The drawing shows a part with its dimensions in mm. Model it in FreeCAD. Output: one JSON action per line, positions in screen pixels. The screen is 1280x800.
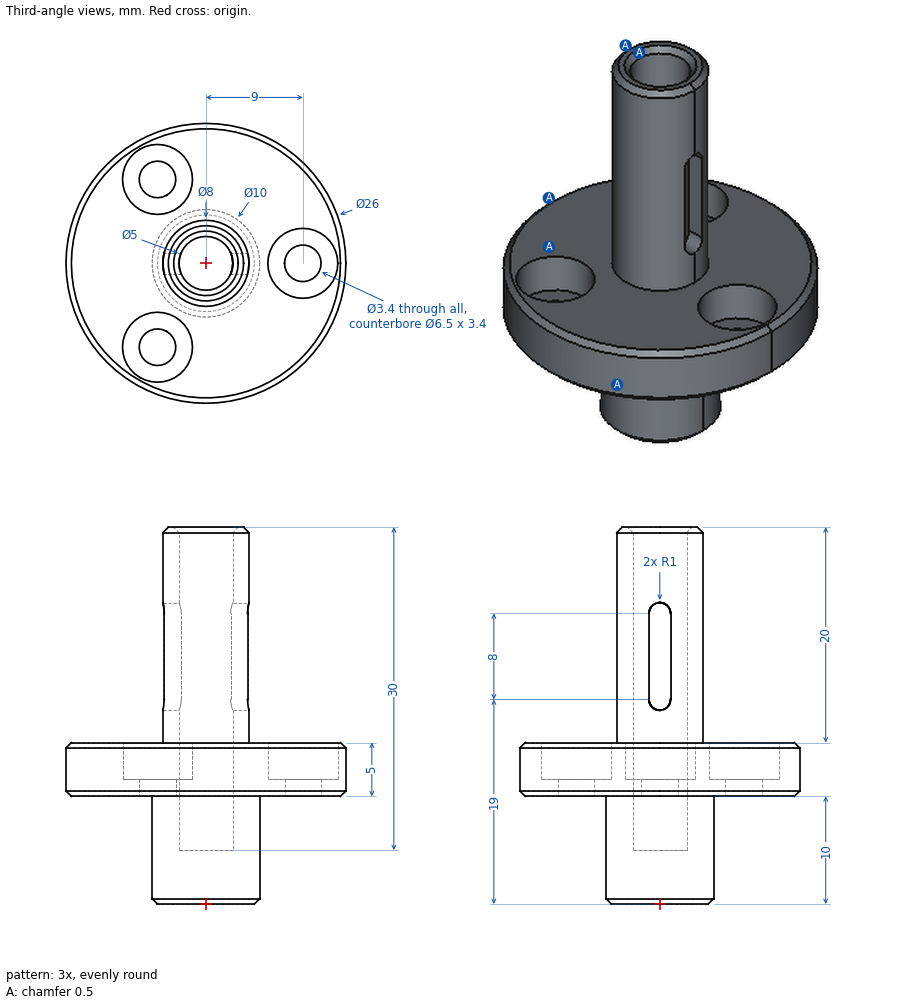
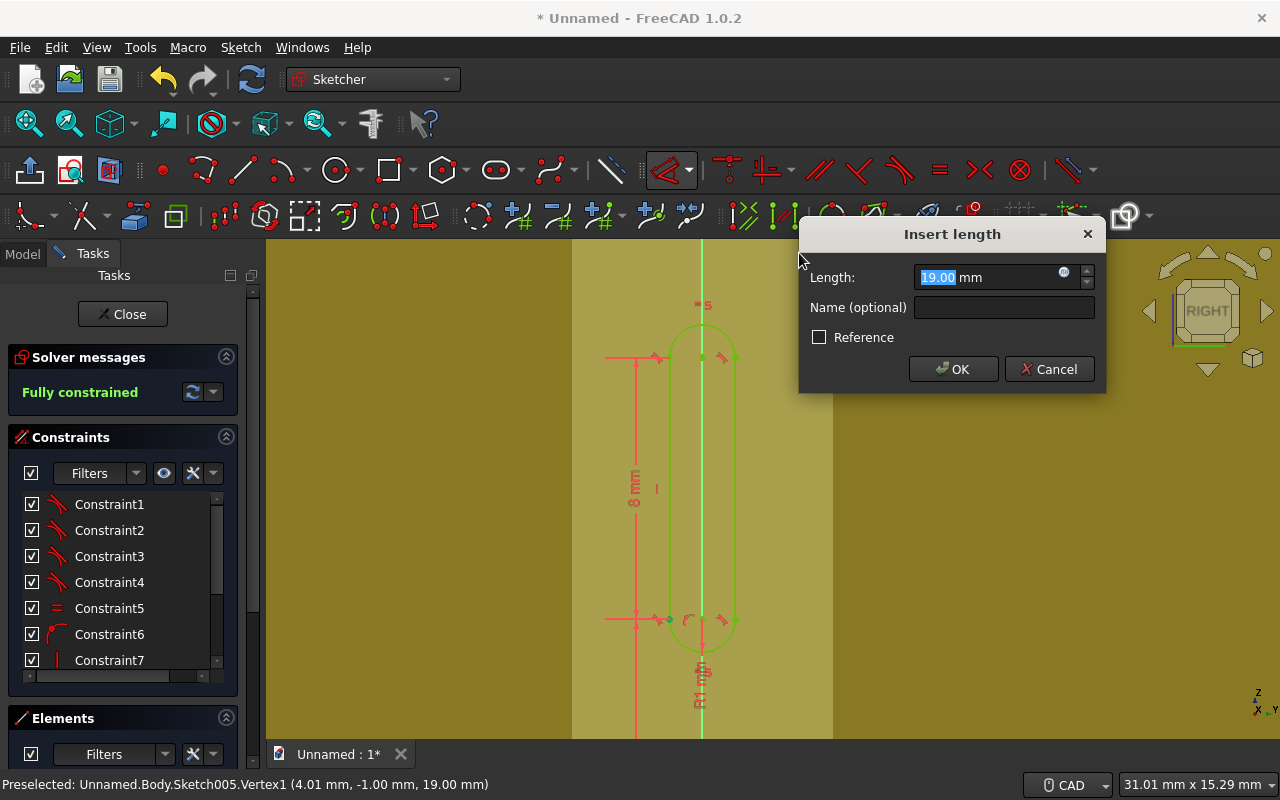
{"action": "type", "text": "19"}
{"action": "key", "text": "Return"}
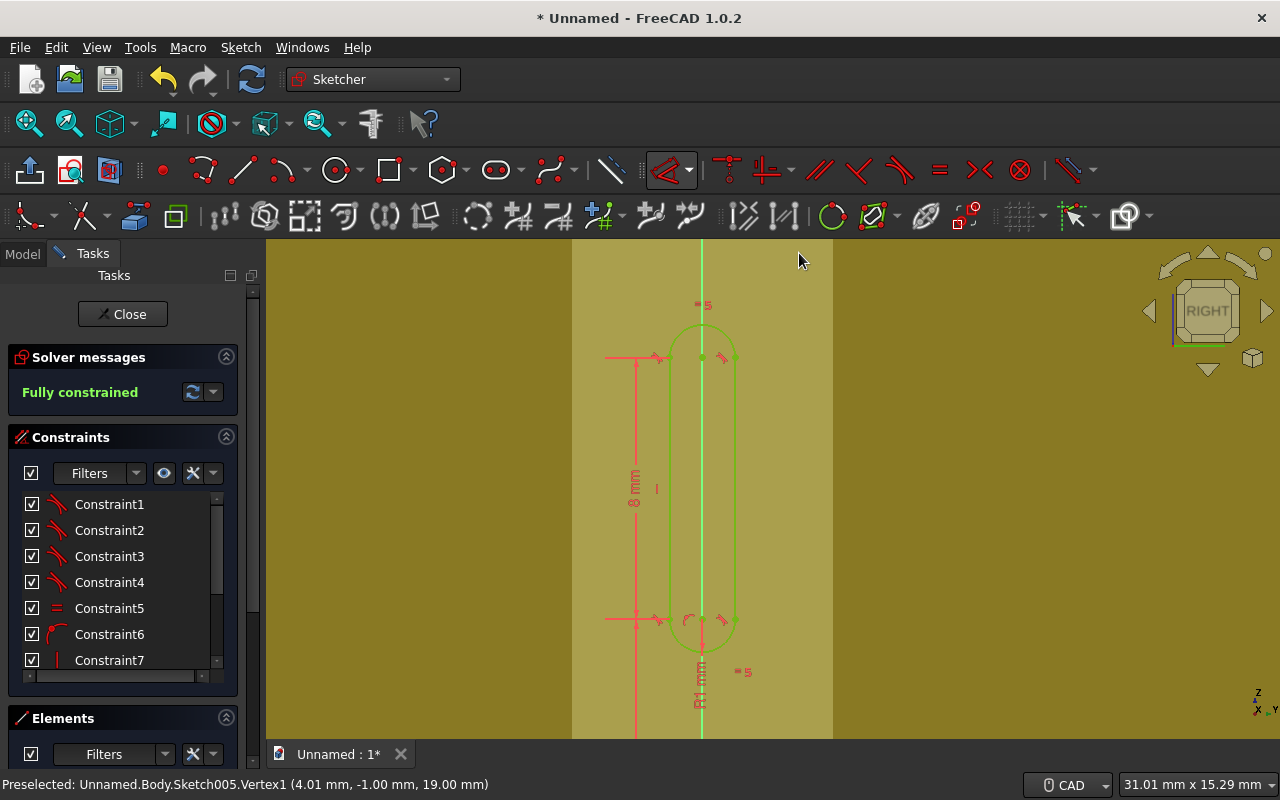
{"action": "left_click", "coordinate": [123, 314]}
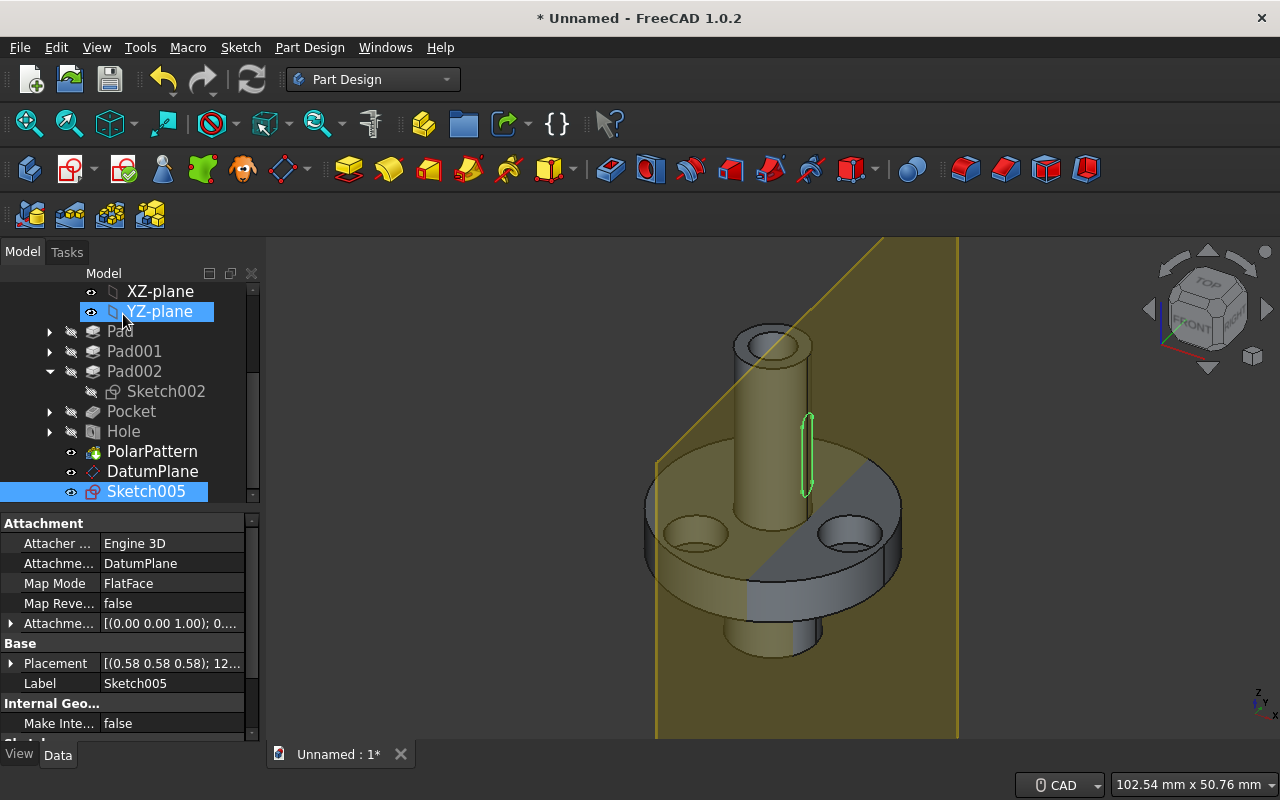
{"action": "left_click", "coordinate": [612, 170]}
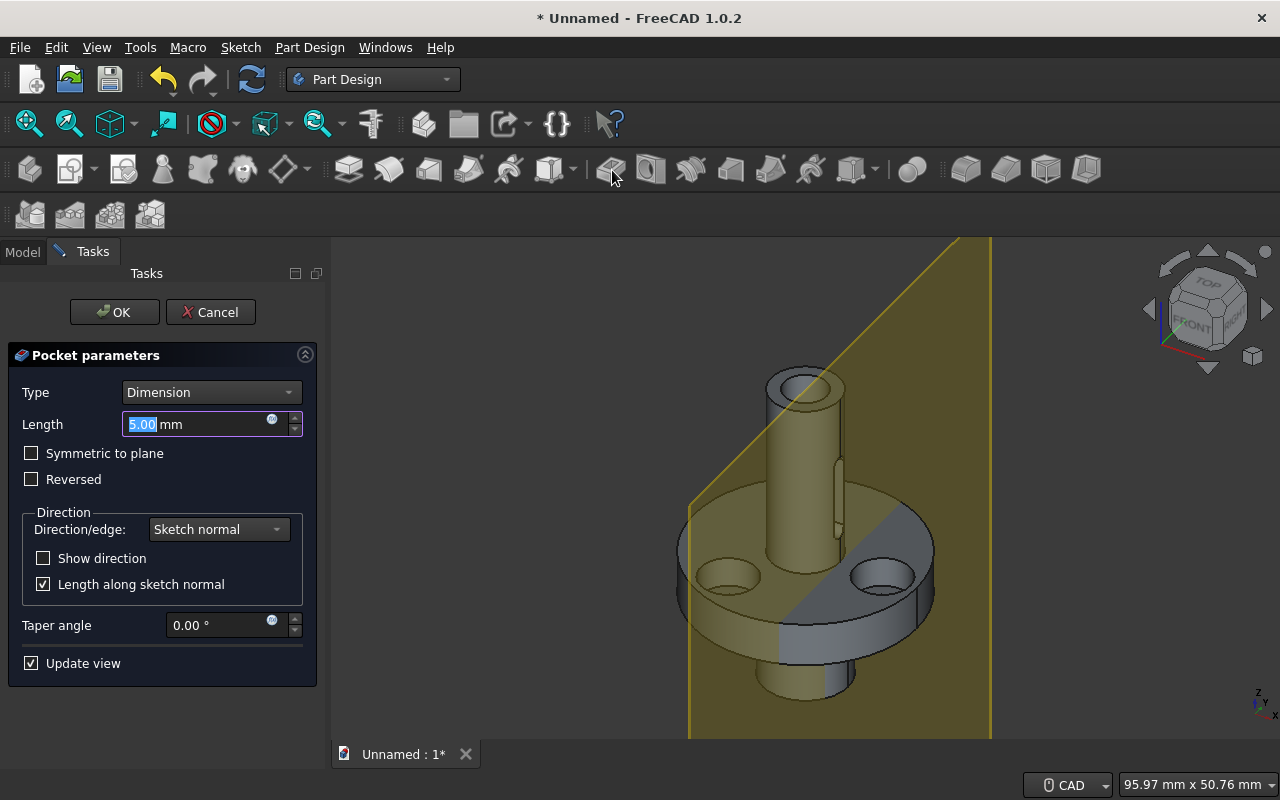
{"action": "left_click", "coordinate": [212, 392]}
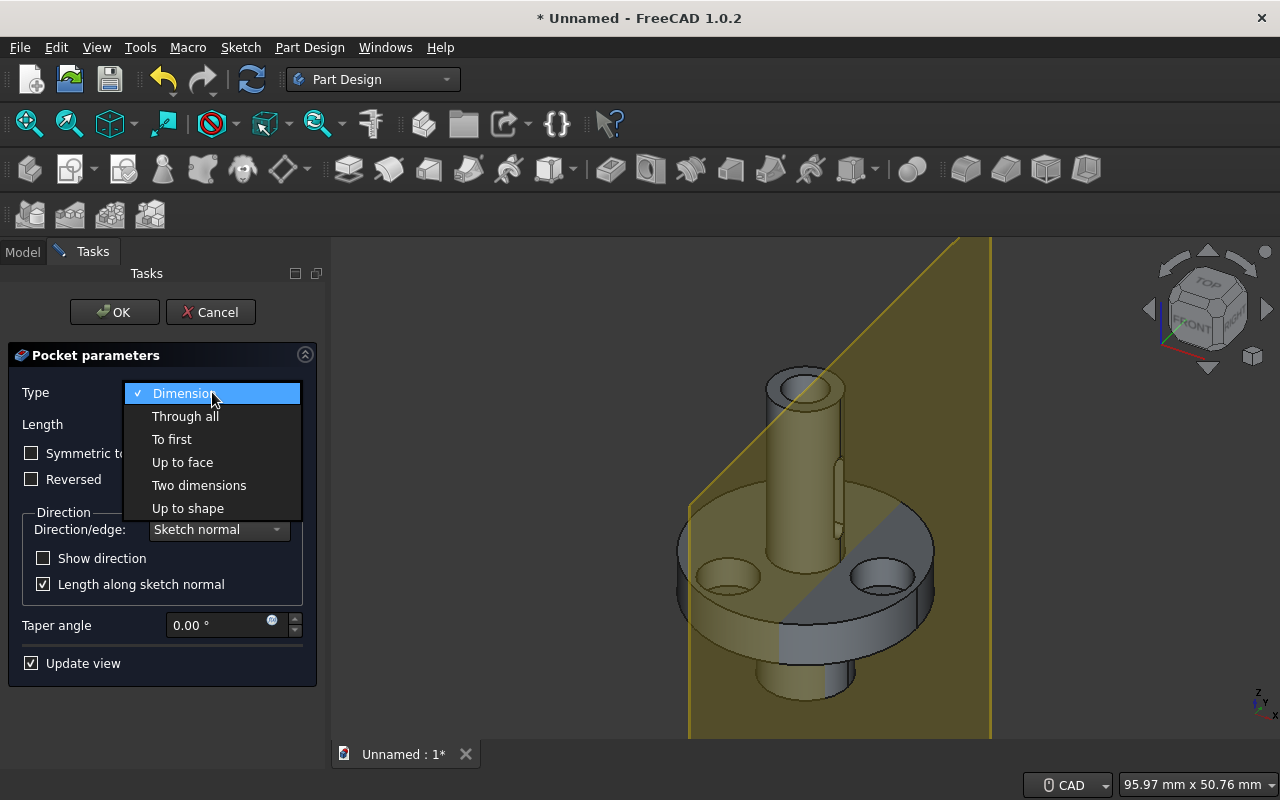
{"action": "left_click", "coordinate": [212, 416]}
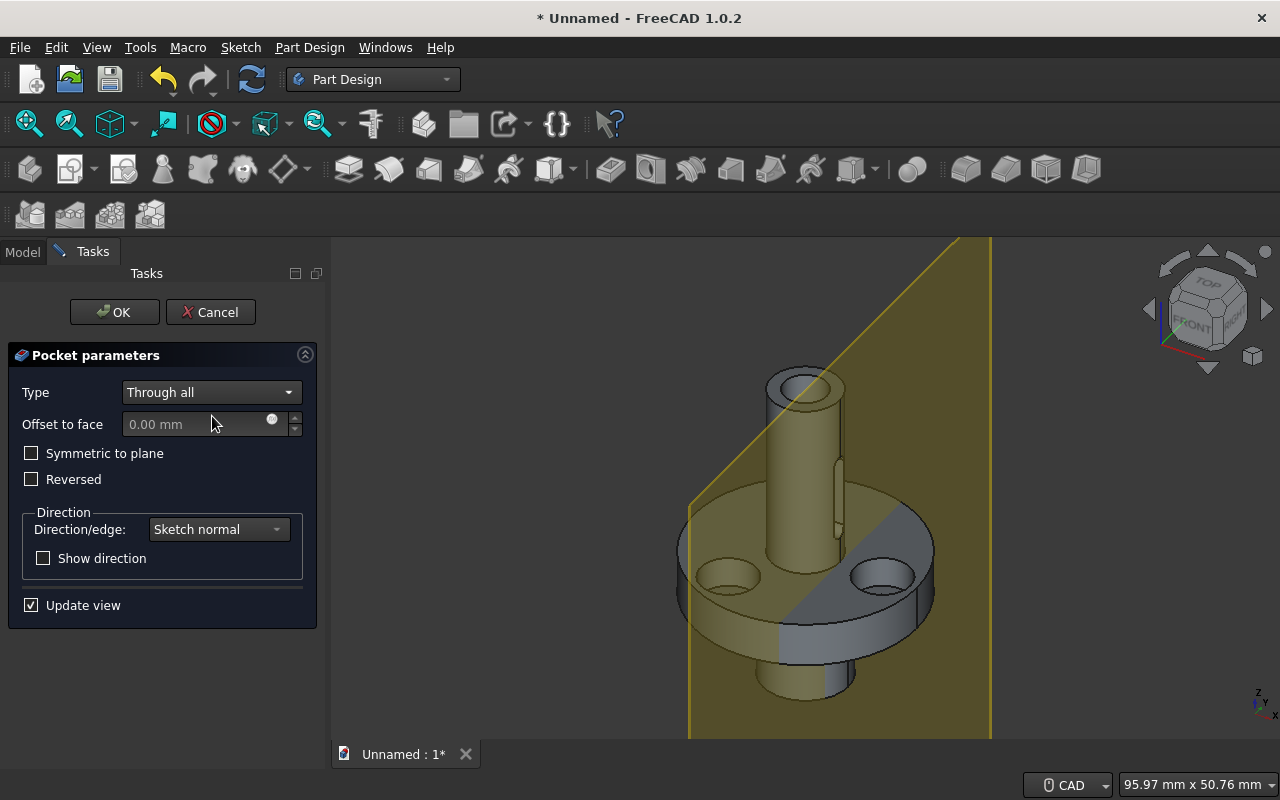
{"action": "left_click", "coordinate": [115, 312]}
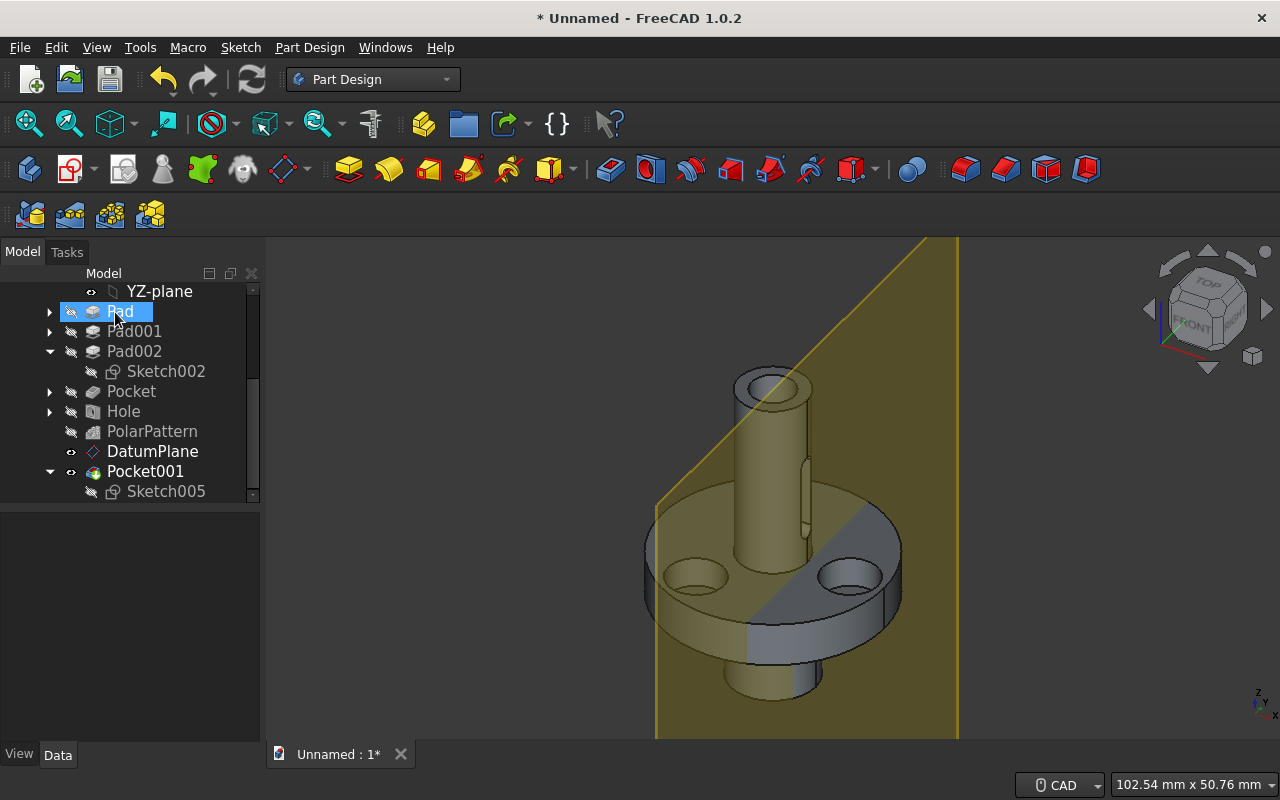
{"action": "left_click", "coordinate": [116, 452]}
{"action": "key", "text": "space"}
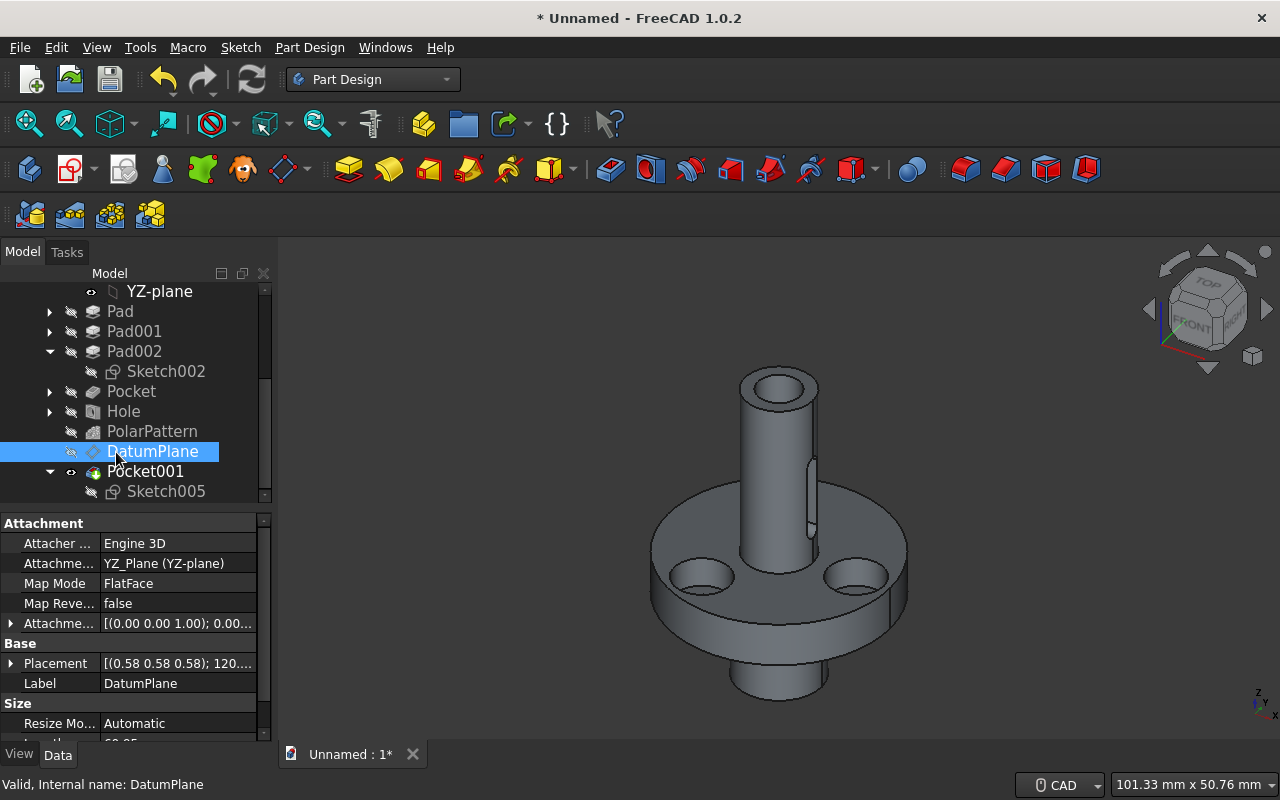
{"action": "left_click", "coordinate": [30, 124]}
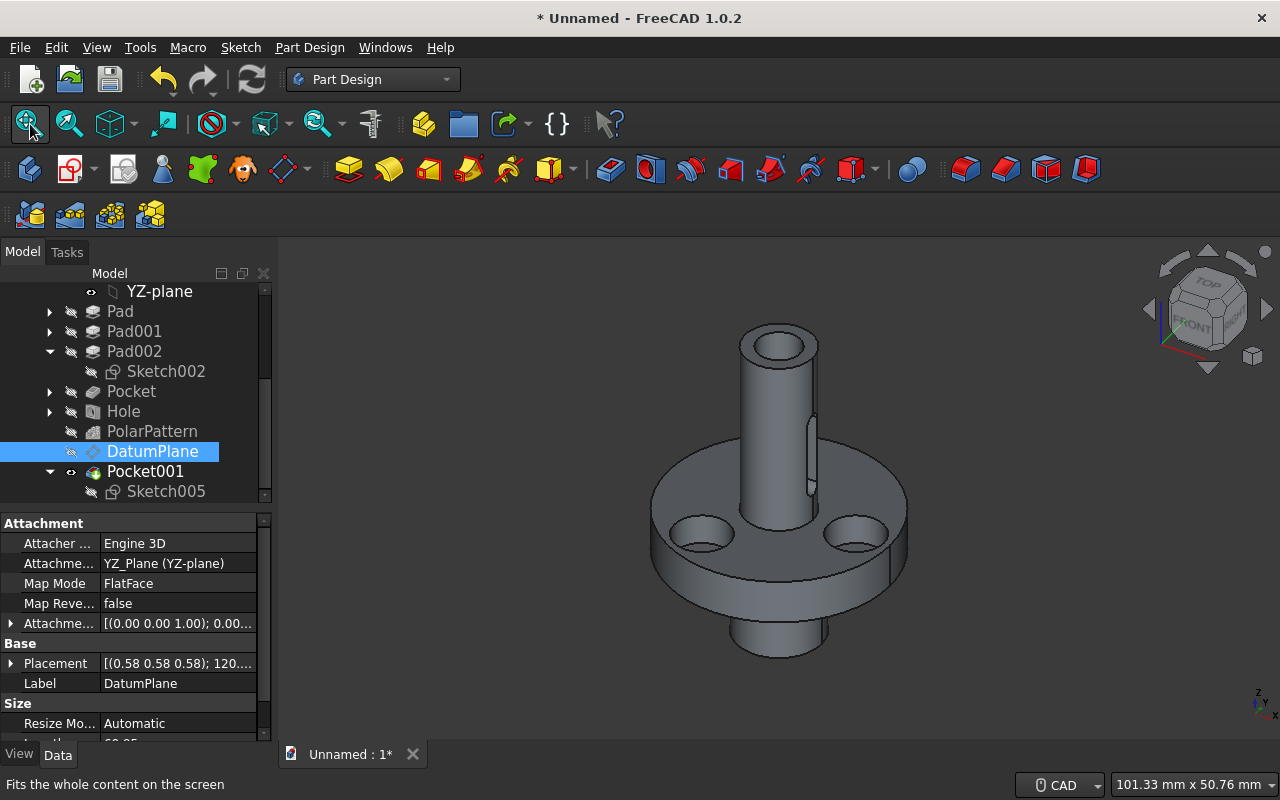
{"action": "left_click", "coordinate": [740, 348]}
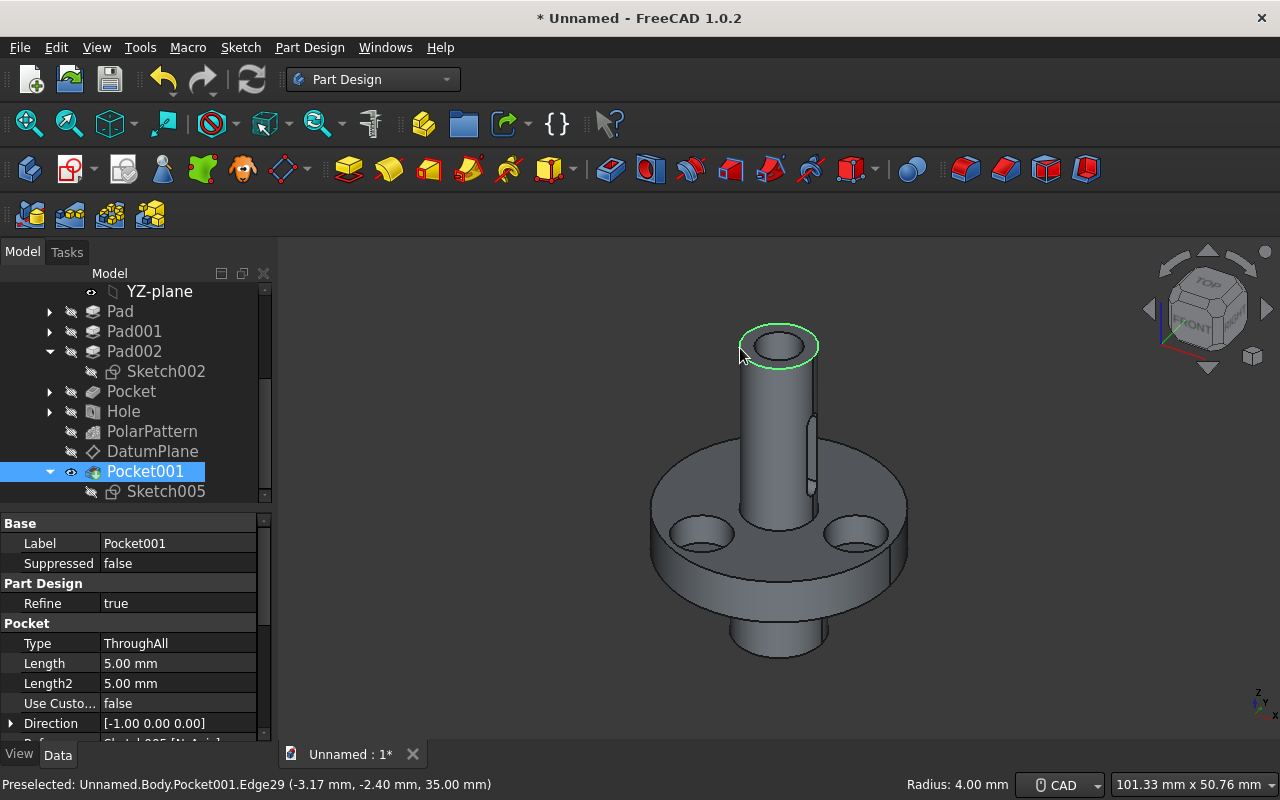
{"action": "left_click", "coordinate": [758, 338], "text": "ctrl"}